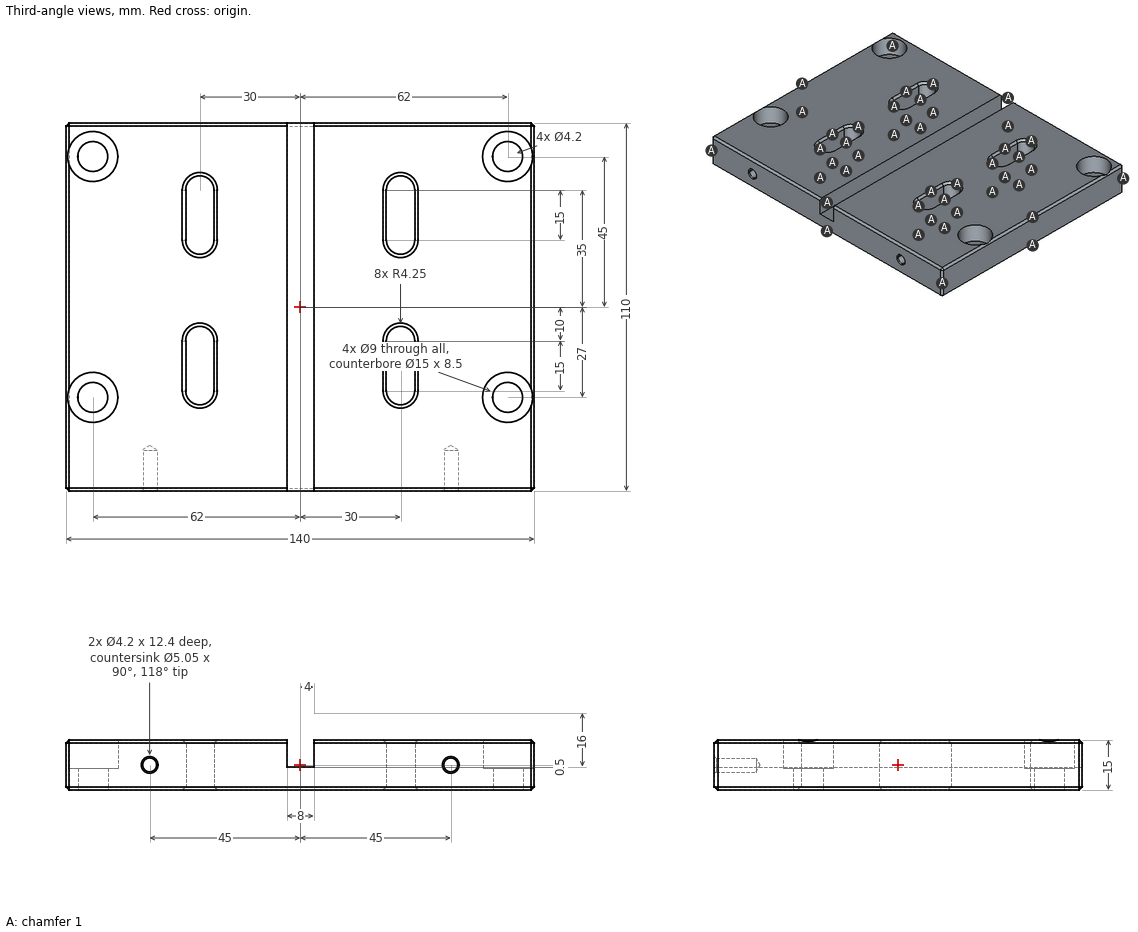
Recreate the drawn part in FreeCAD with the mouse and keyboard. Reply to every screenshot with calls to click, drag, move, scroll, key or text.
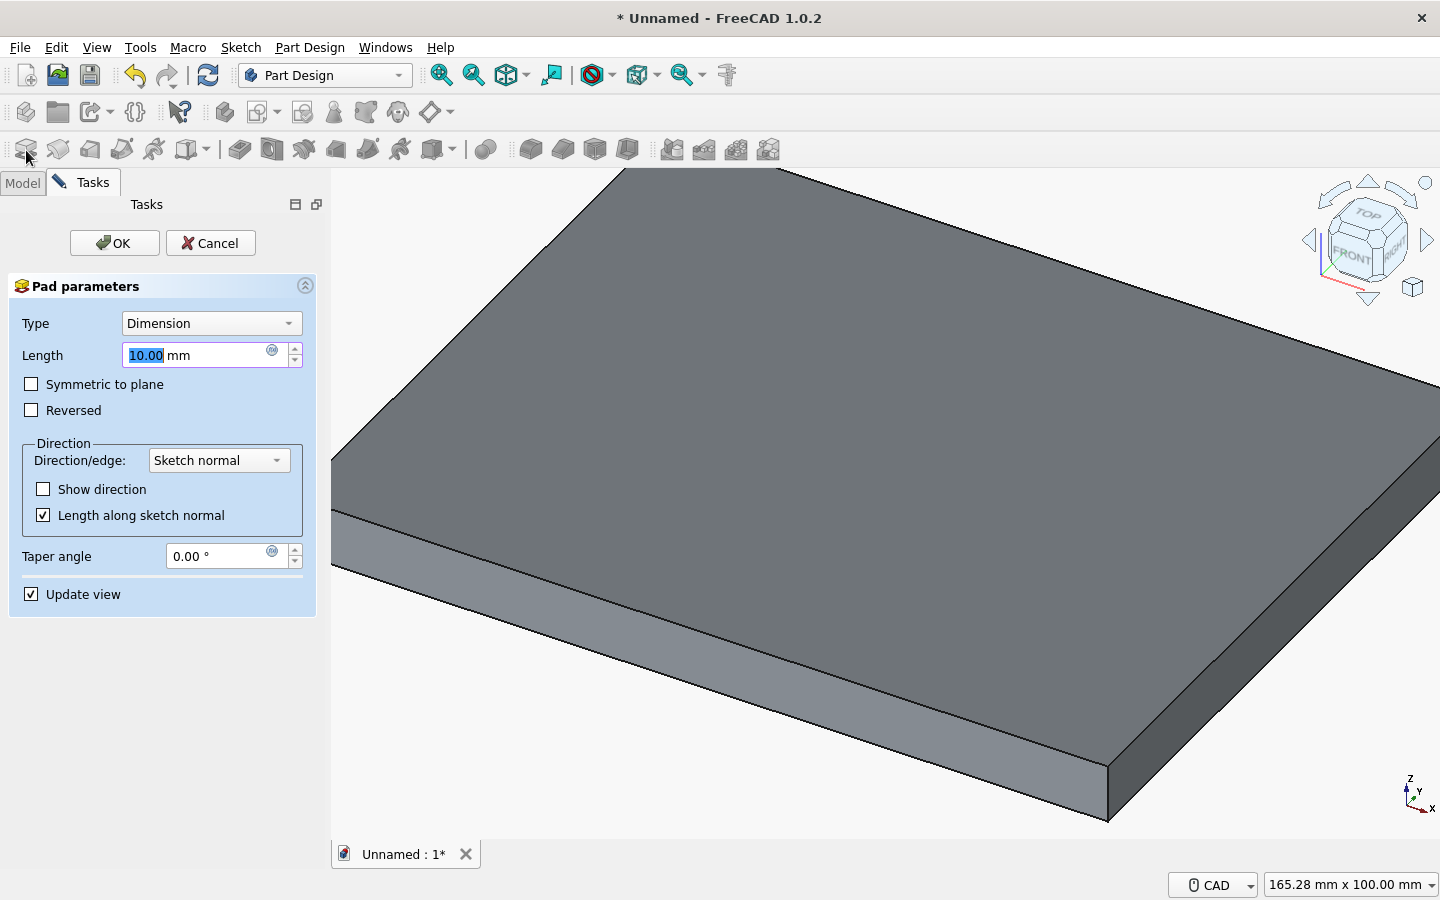
text(15)
key(Tab)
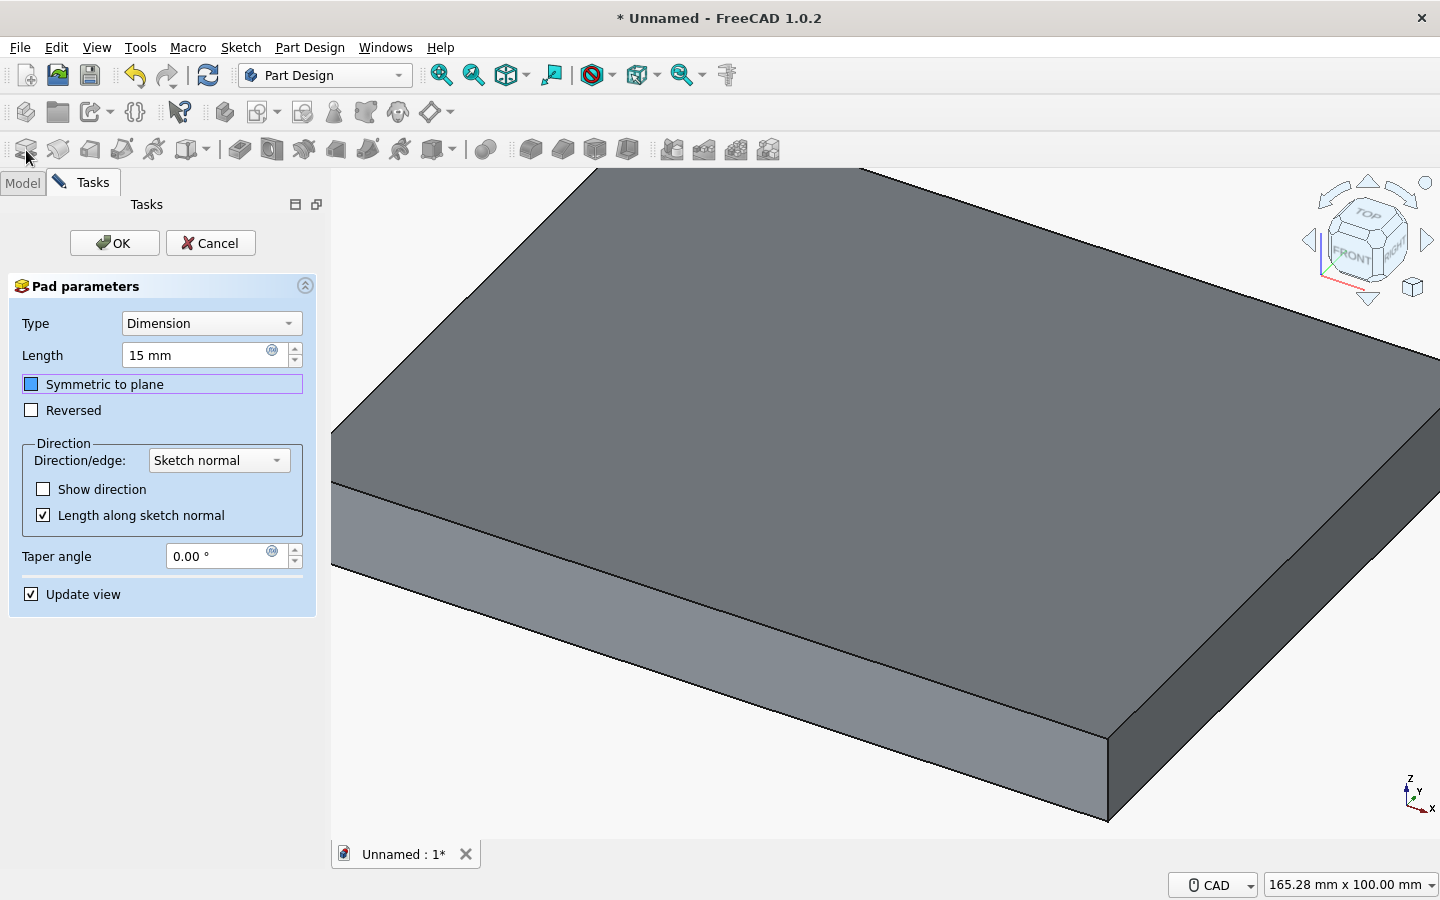
click(30, 384)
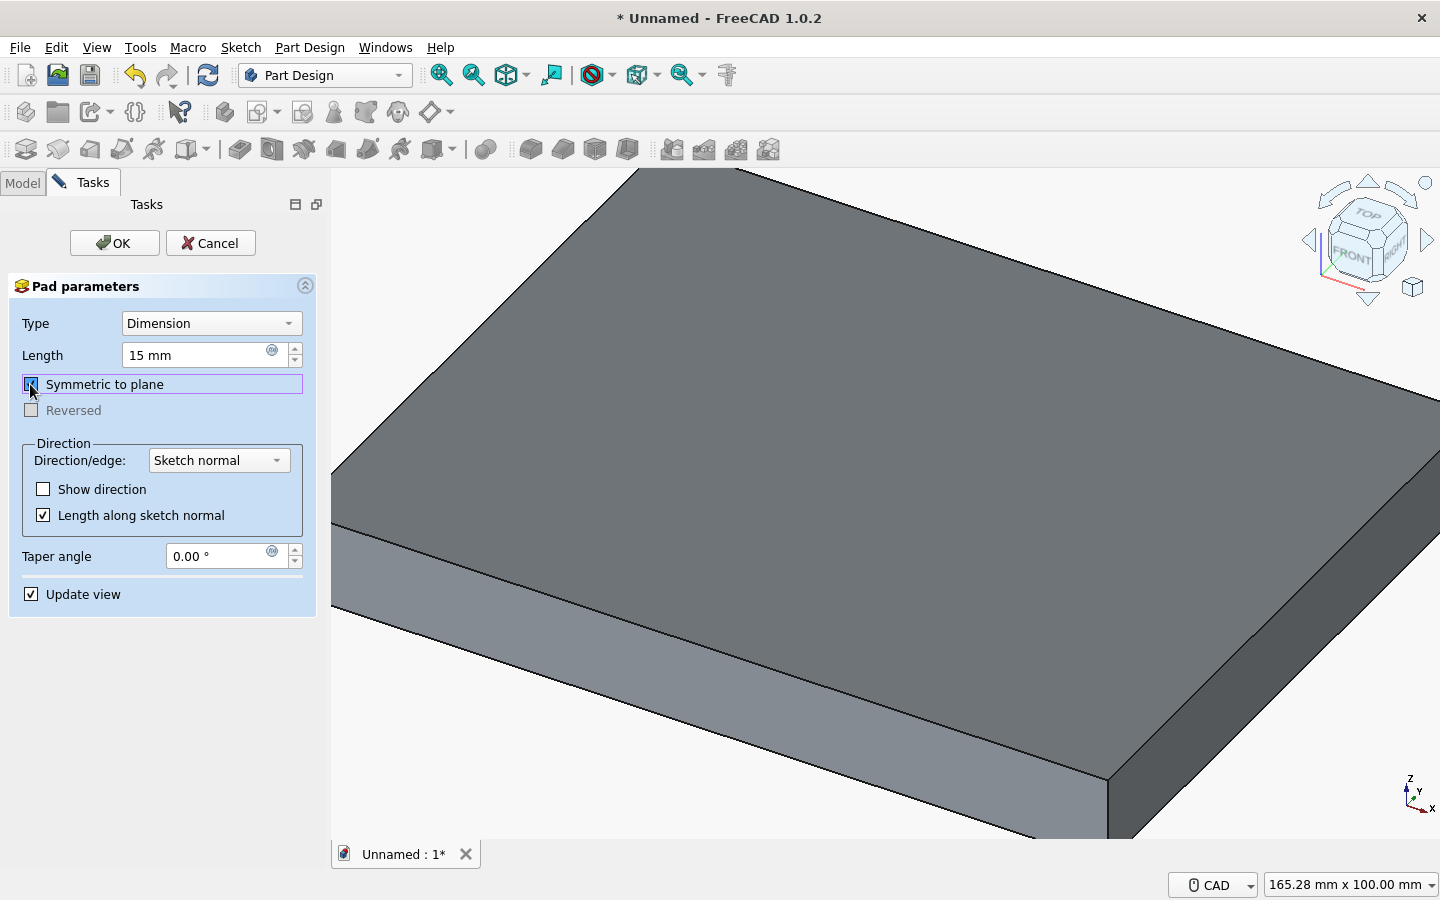
click(115, 243)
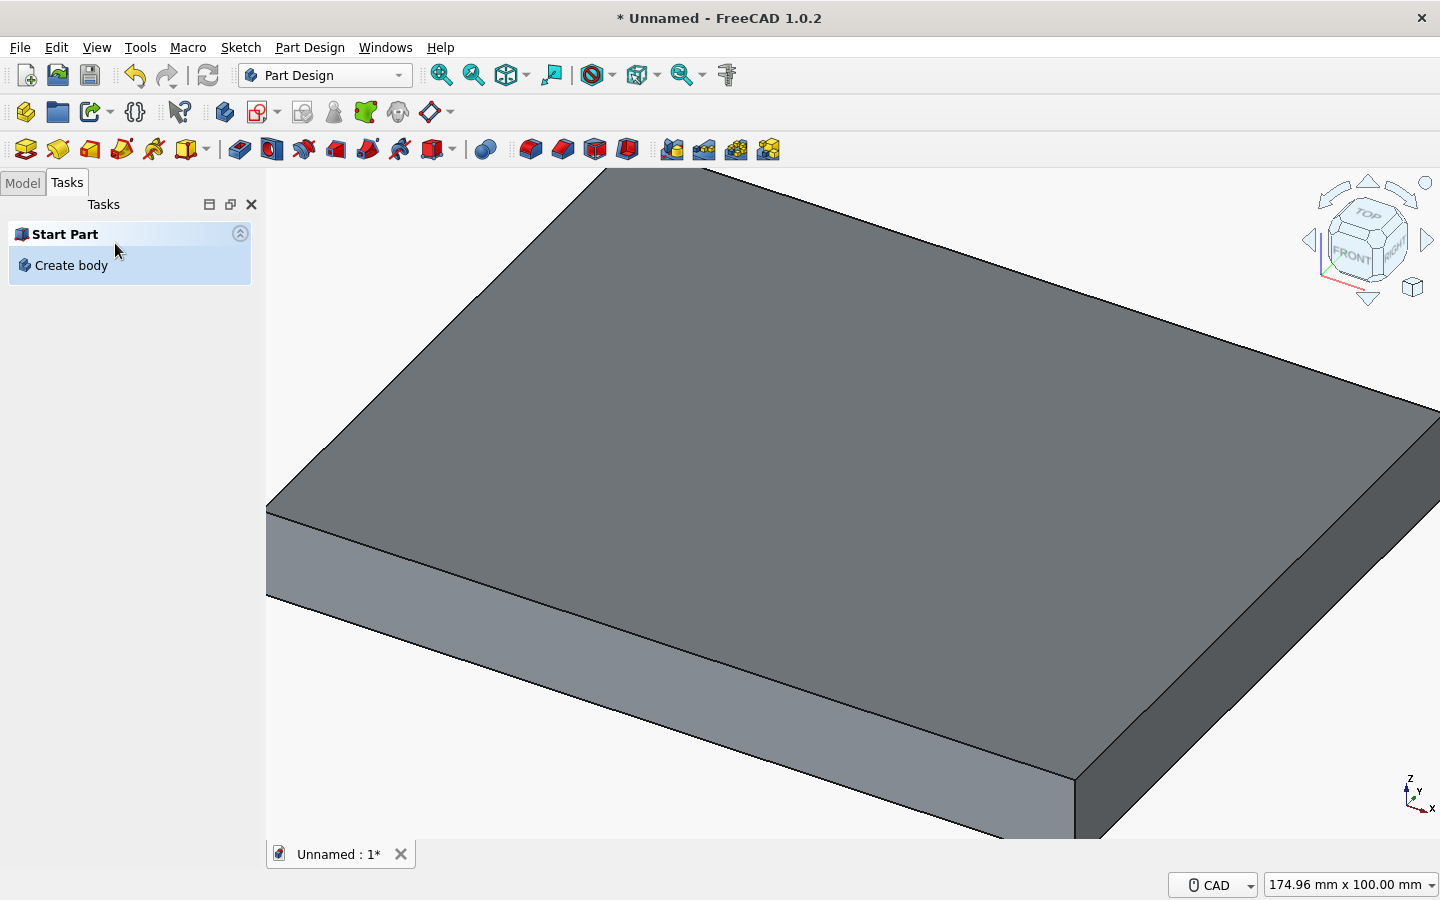
click(442, 76)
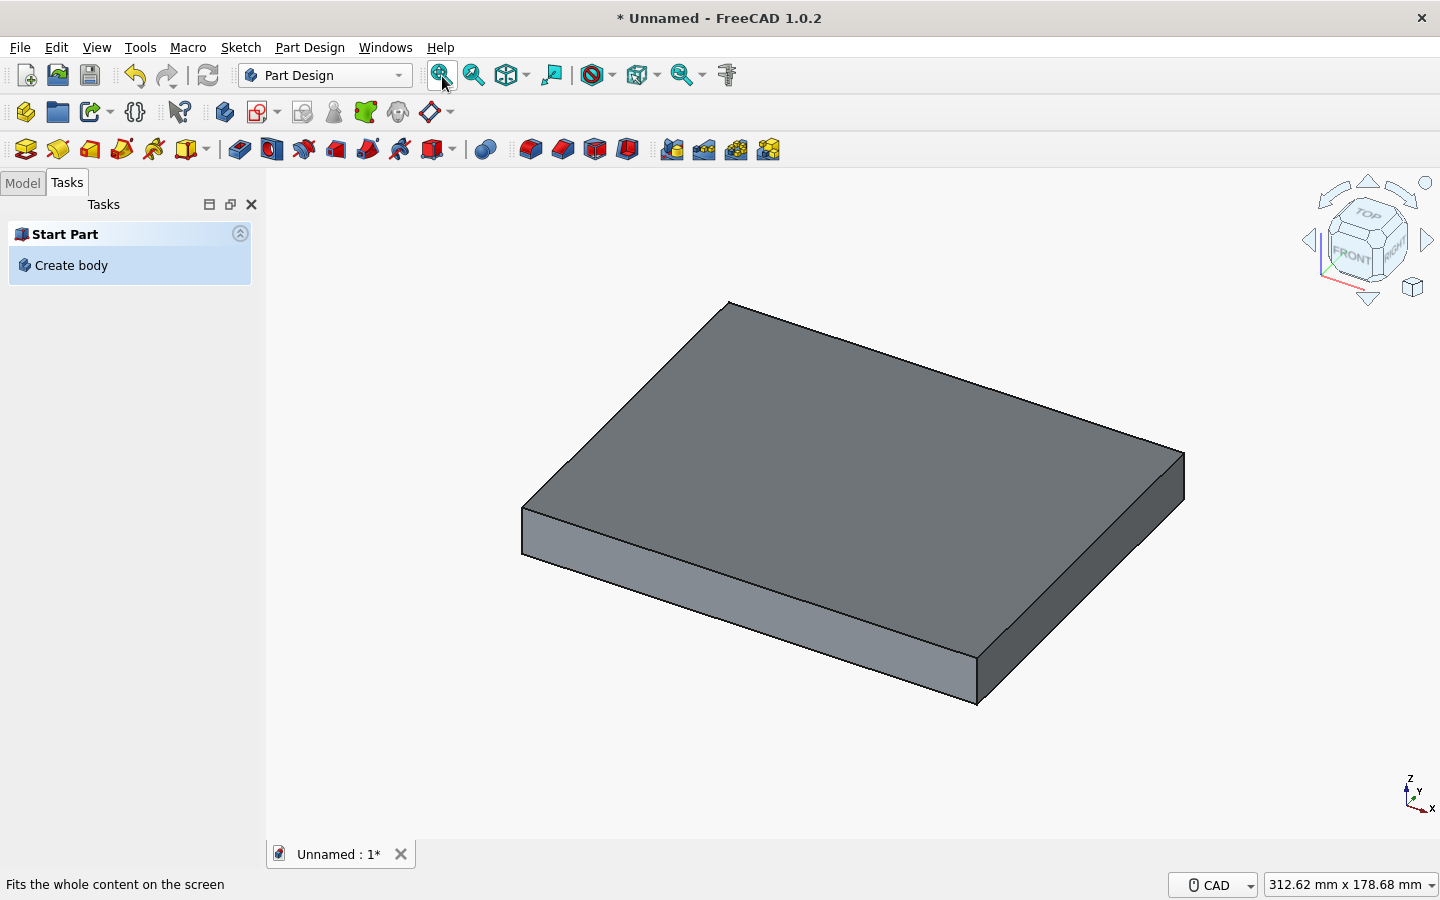
key(5)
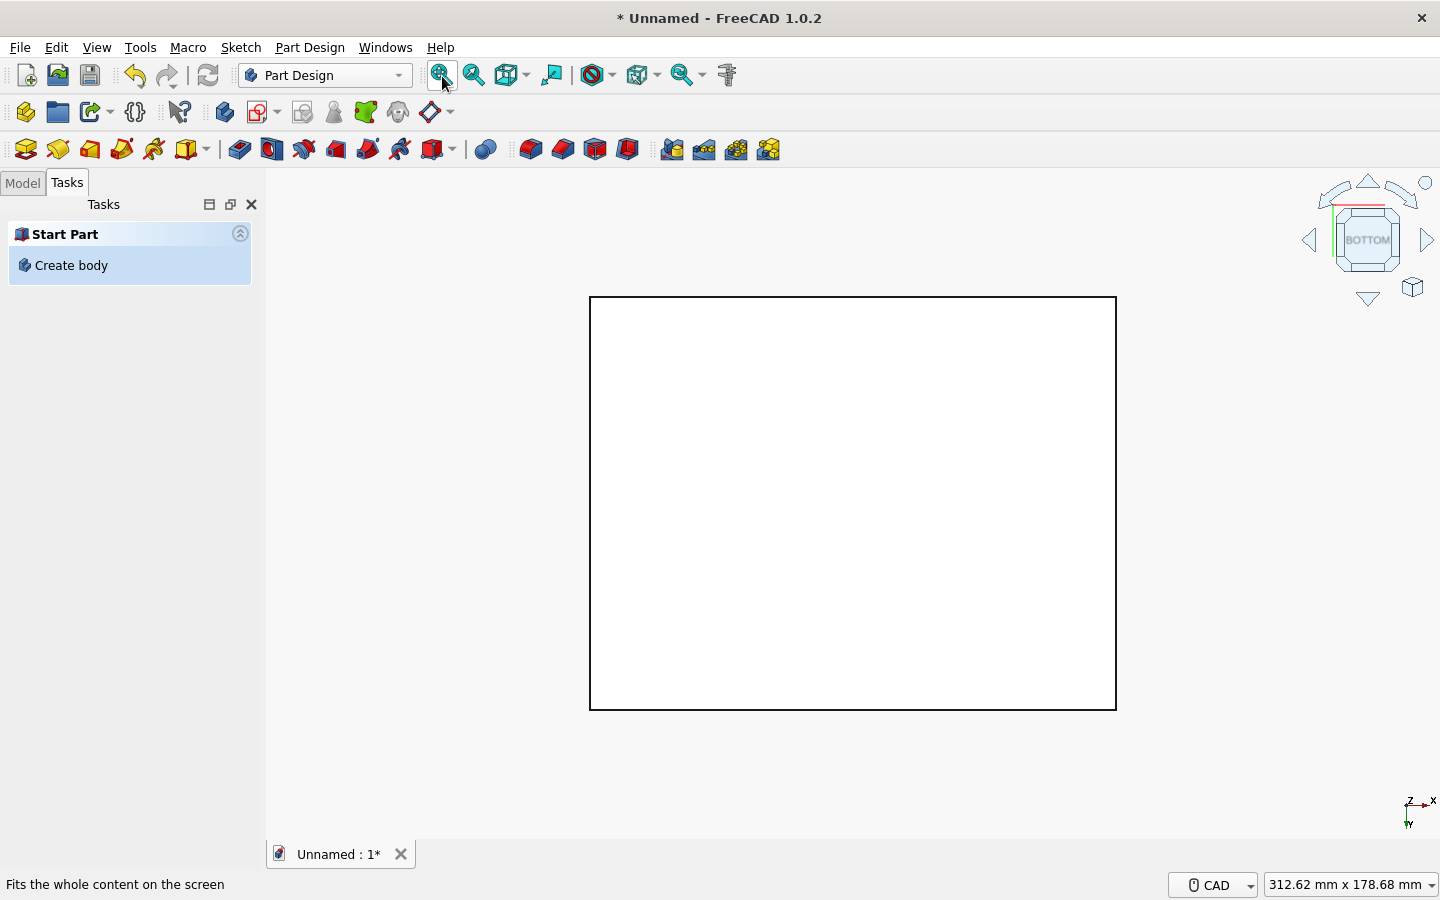
click(853, 502)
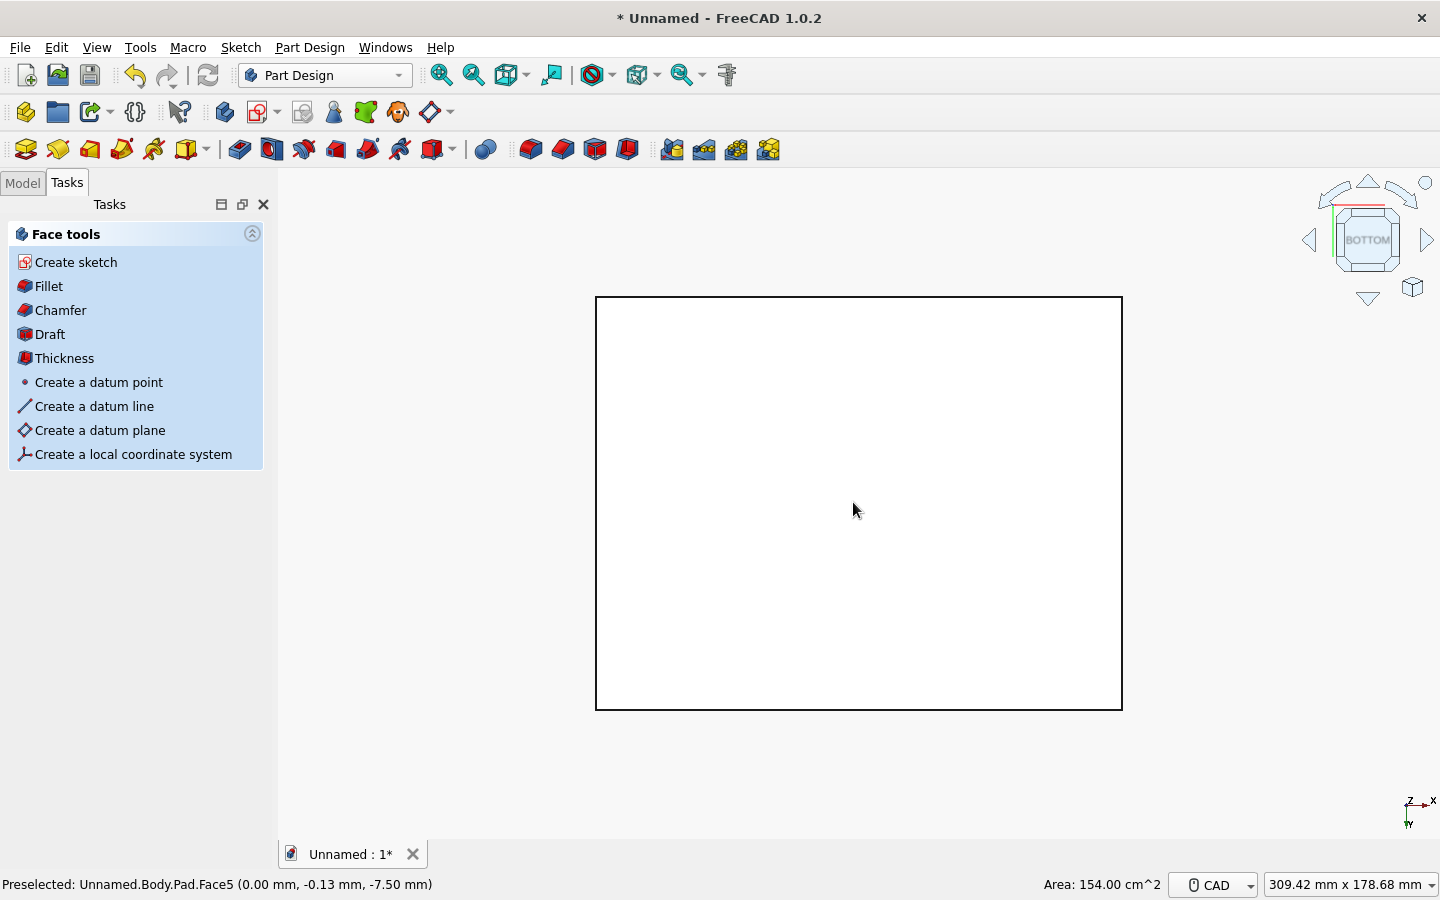
click(258, 112)